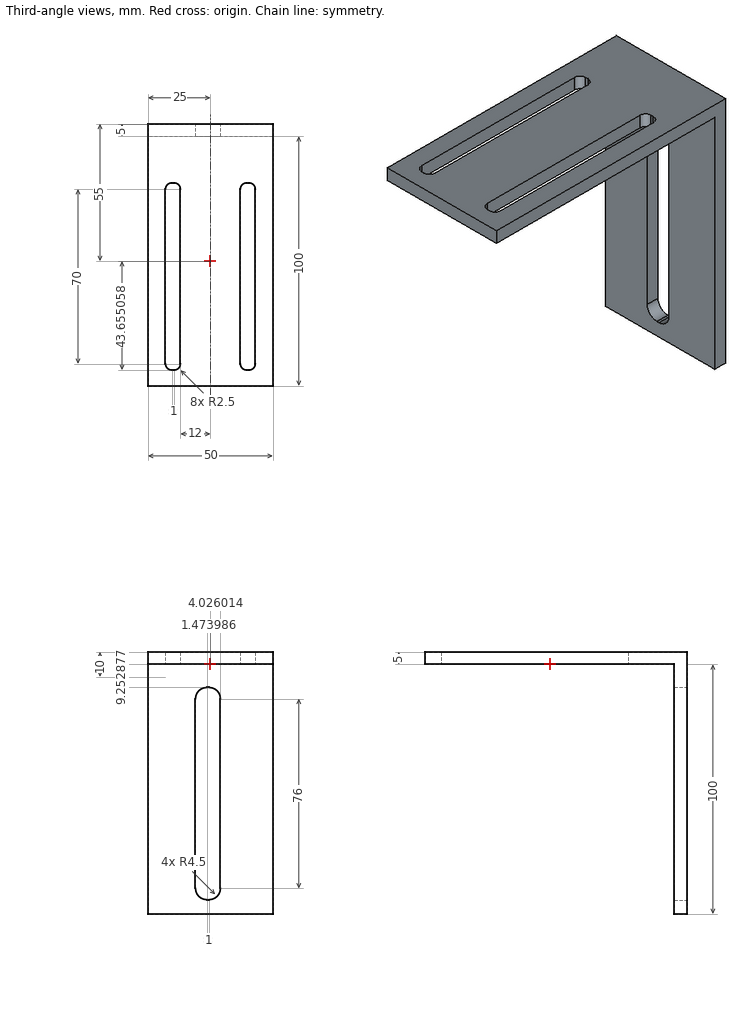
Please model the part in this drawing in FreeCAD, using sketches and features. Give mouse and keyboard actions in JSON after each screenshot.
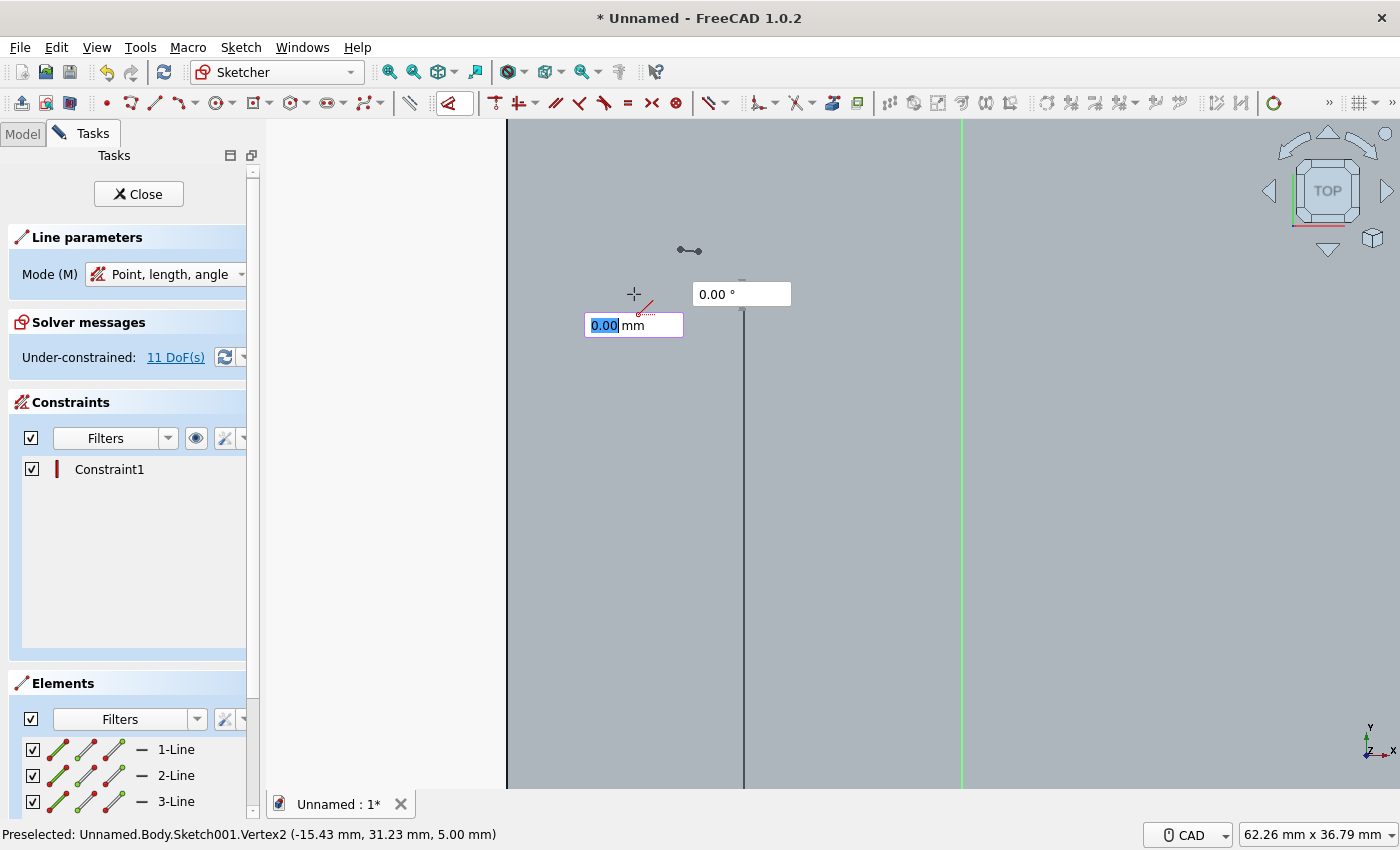
{"action": "scroll", "coordinate": [679, 248], "scroll_direction": "down", "scroll_amount": 6}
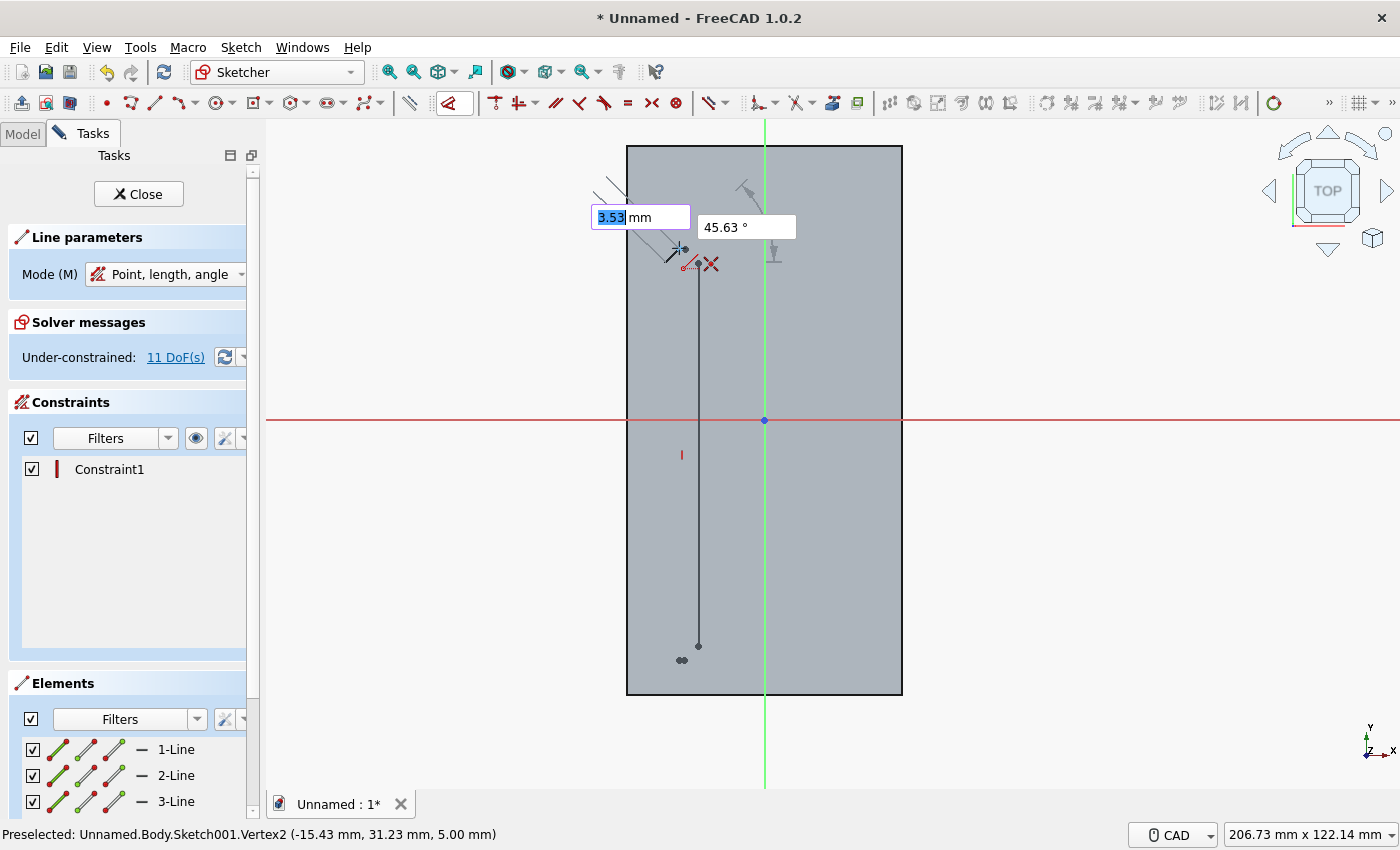
{"action": "left_click", "coordinate": [666, 646]}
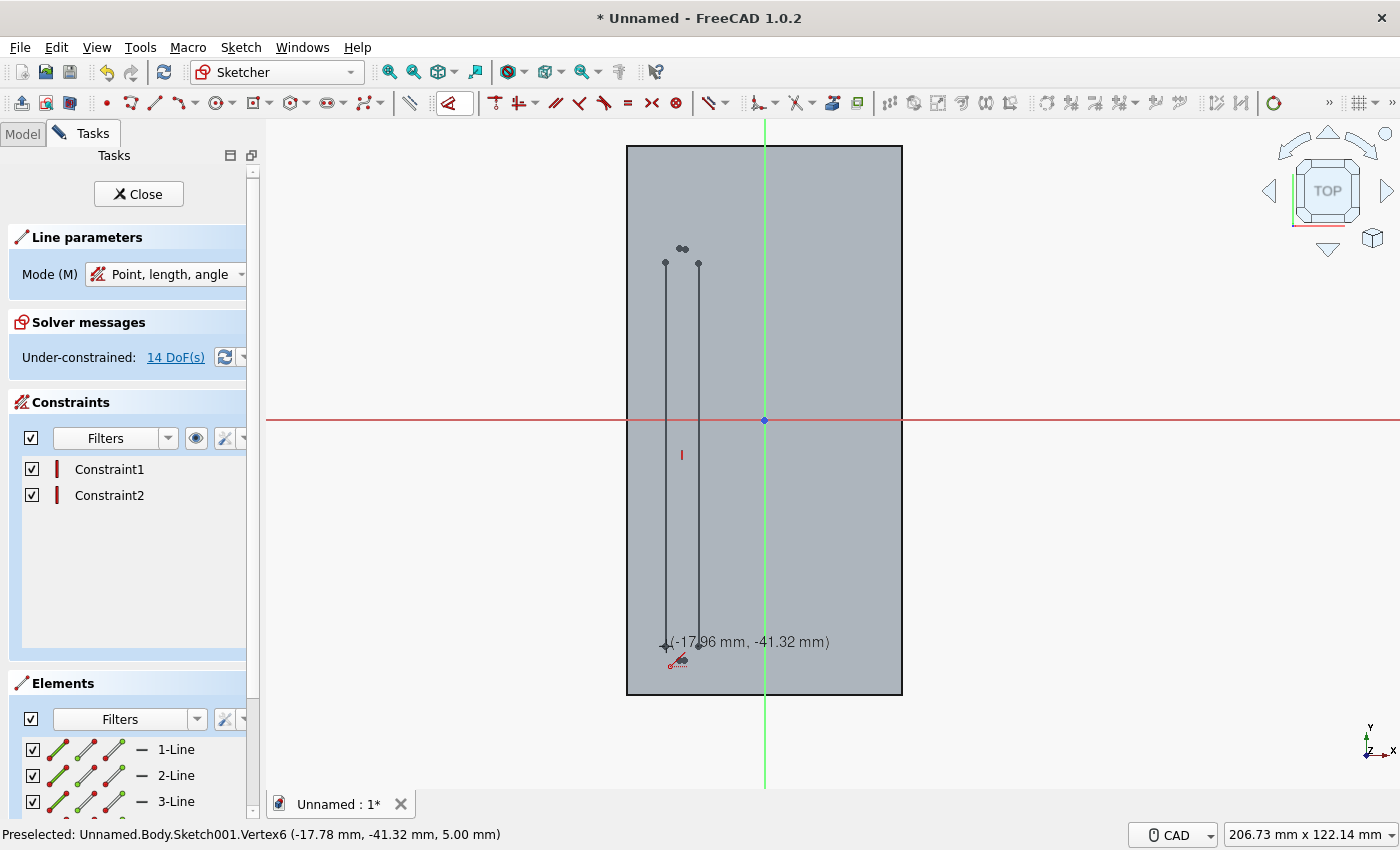
{"action": "key", "text": "g 3 a"}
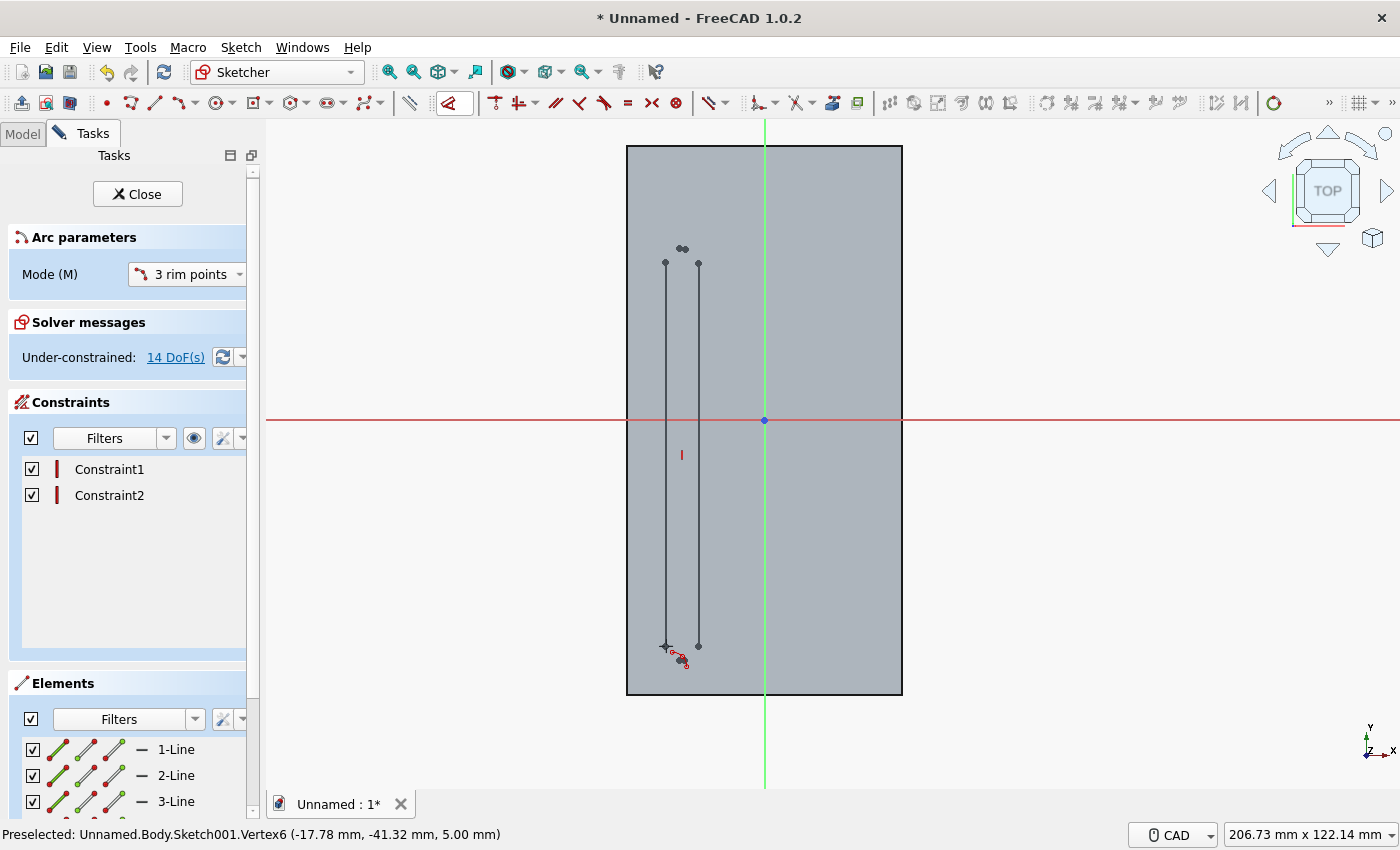
{"action": "scroll", "coordinate": [685, 660], "scroll_direction": "up", "scroll_amount": 9}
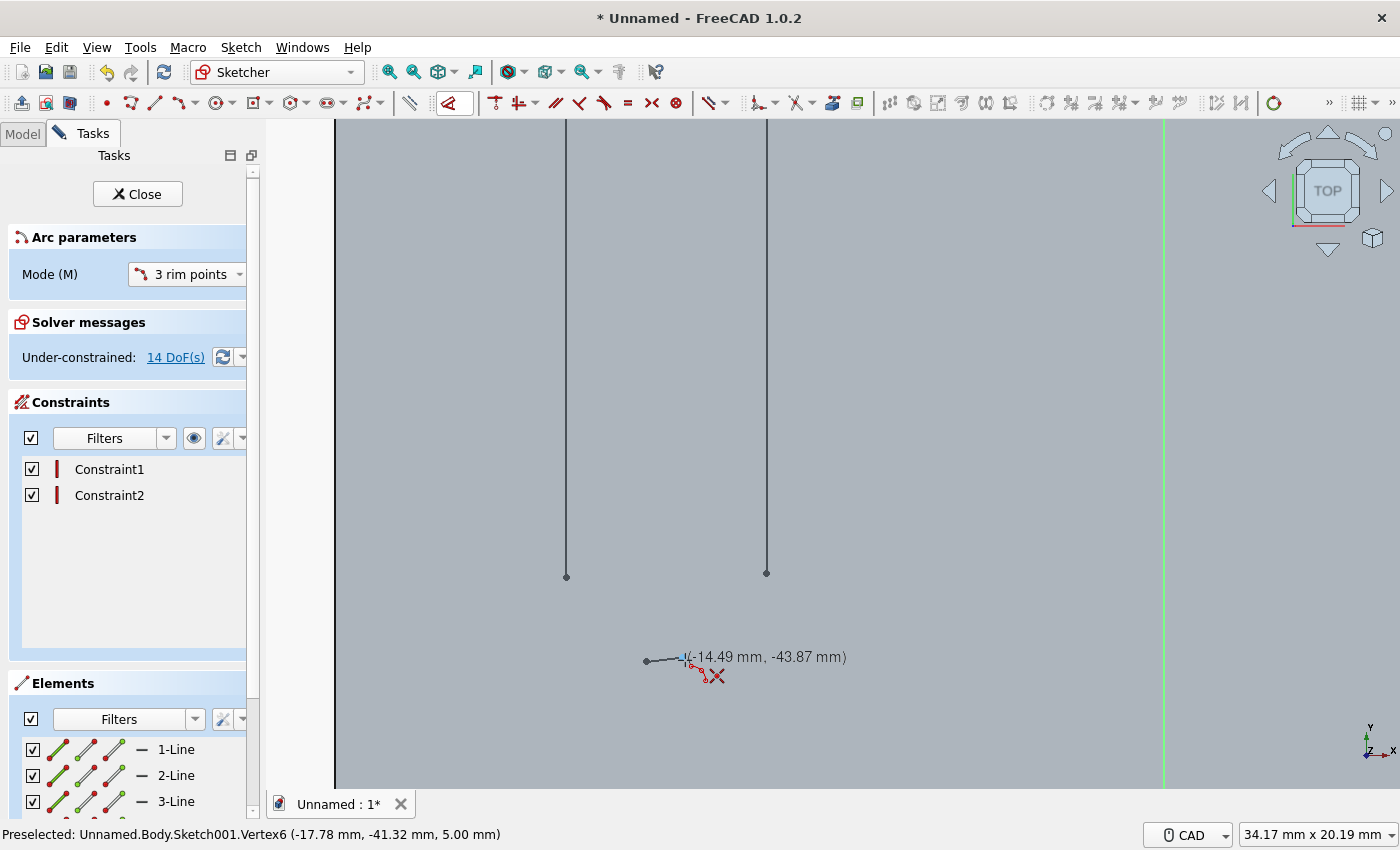
{"action": "left_click", "coordinate": [683, 658]}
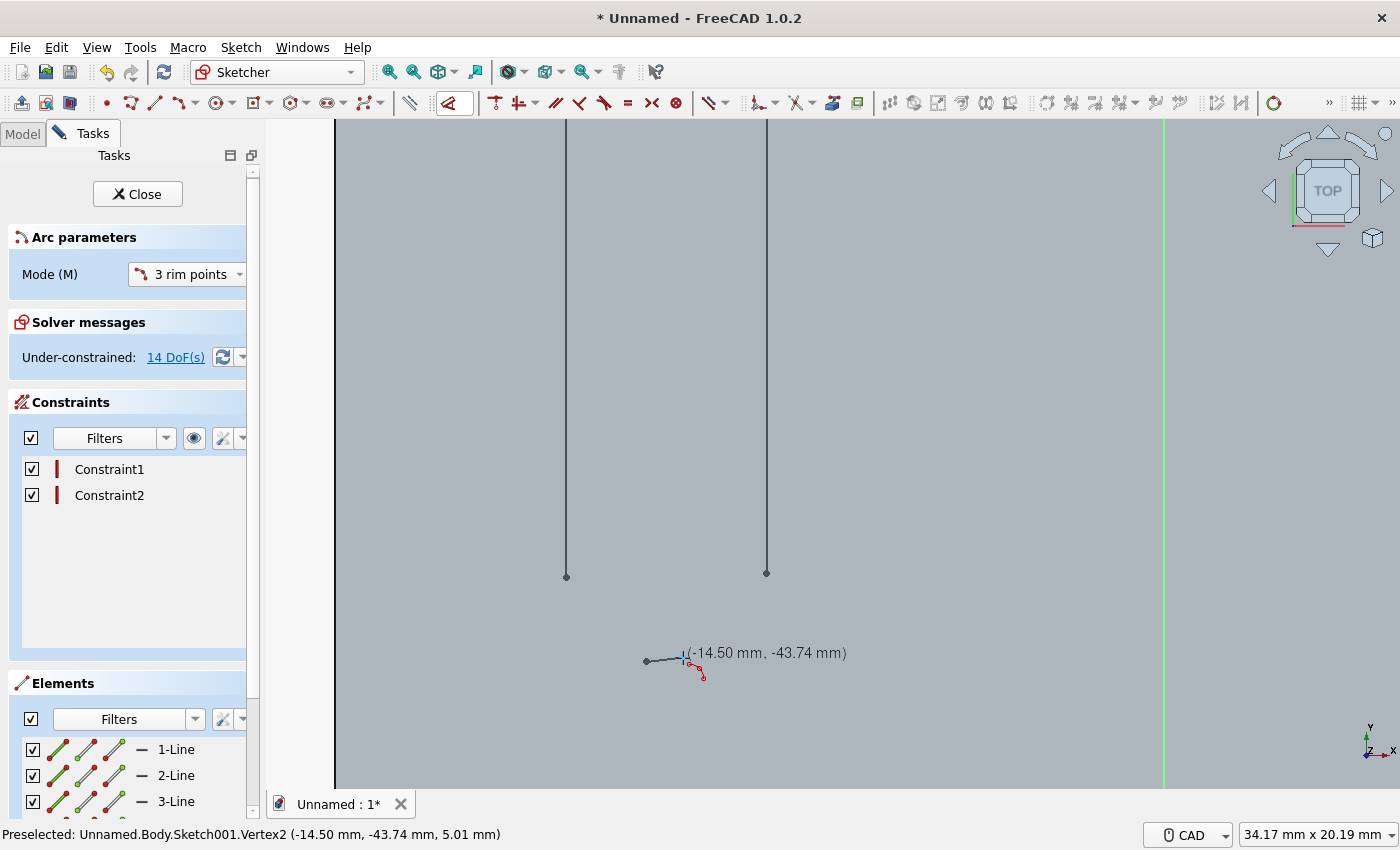
{"action": "scroll", "coordinate": [685, 661], "scroll_direction": "down", "scroll_amount": 9}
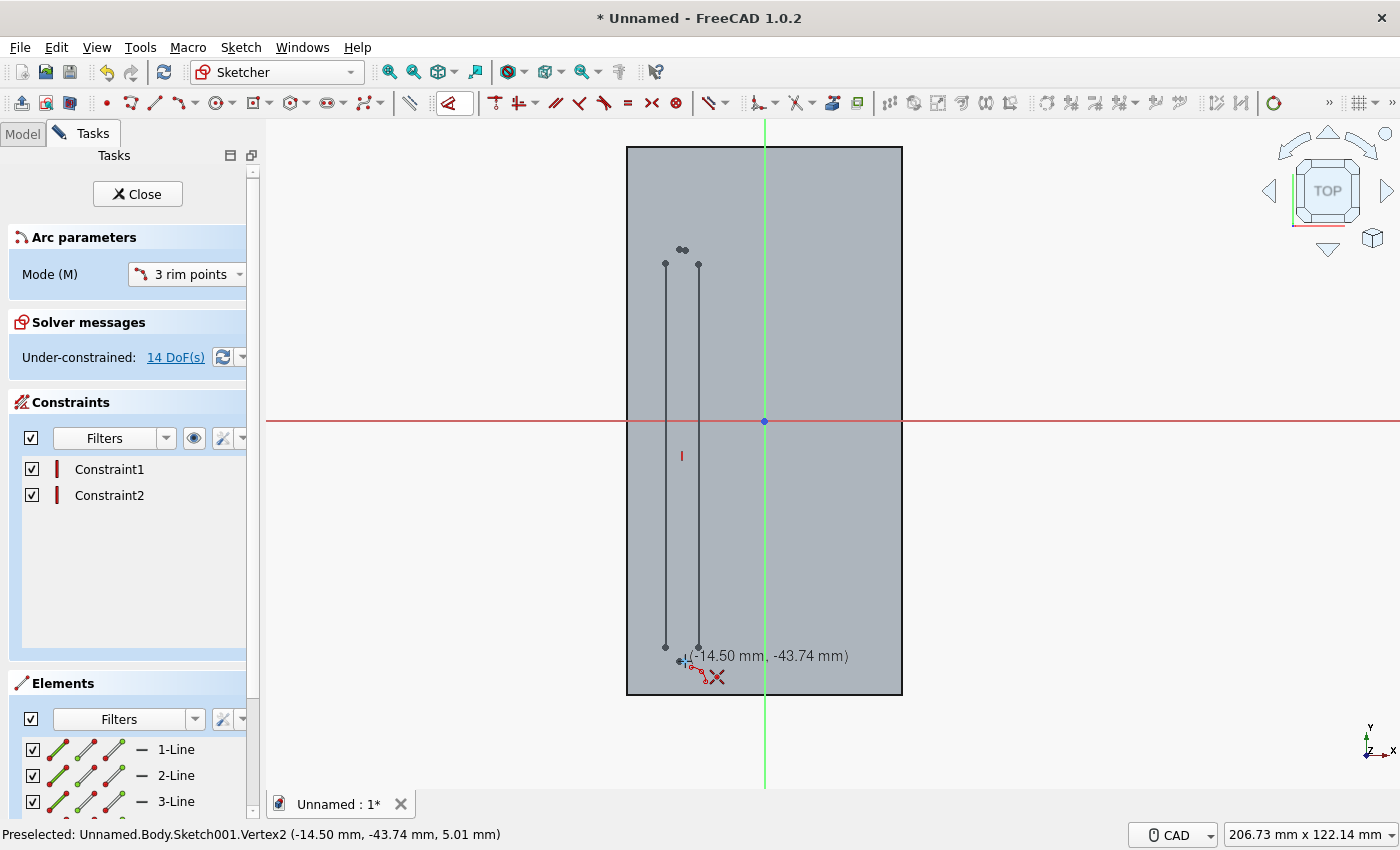
{"action": "left_click", "coordinate": [699, 647]}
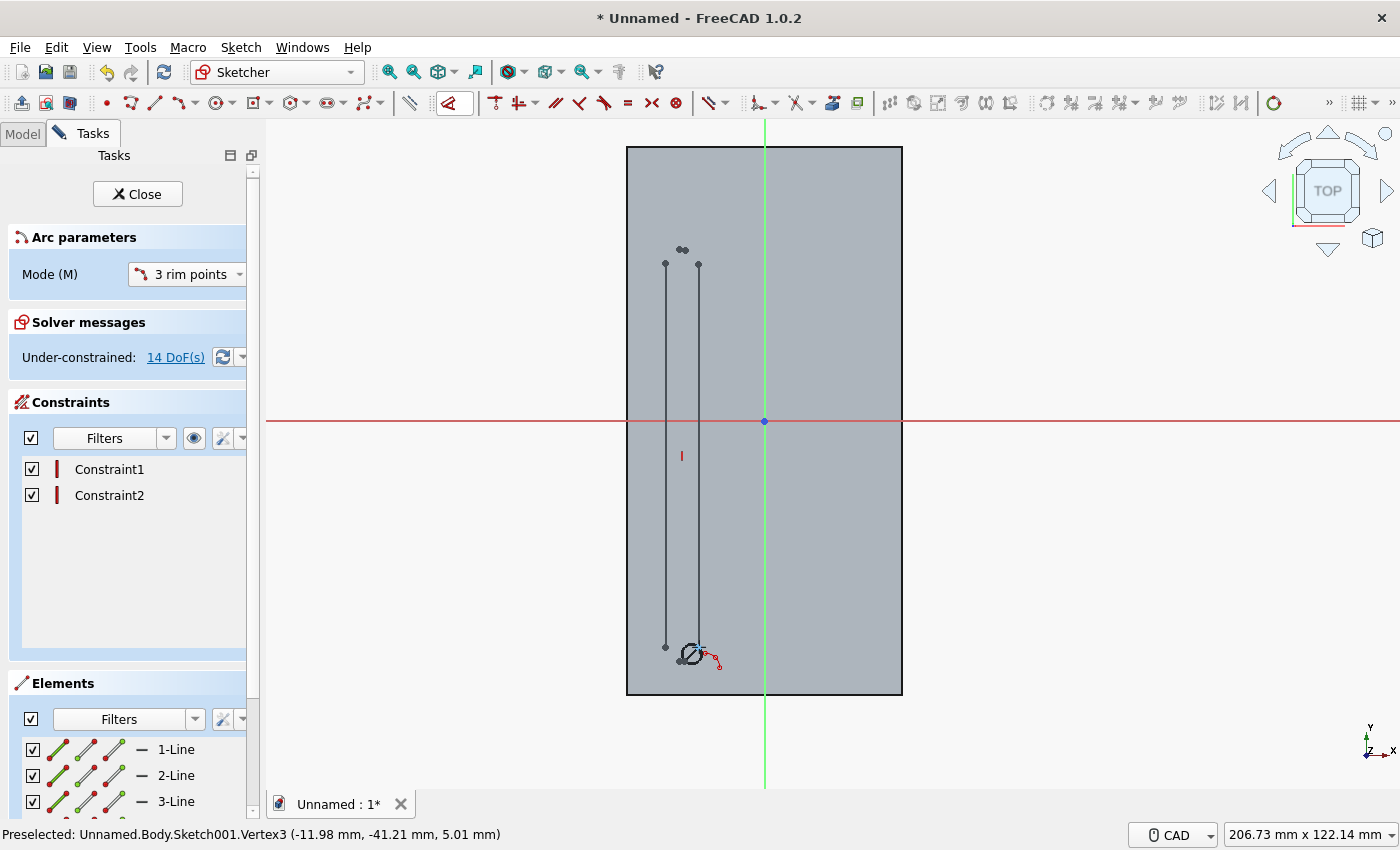
{"action": "scroll", "coordinate": [695, 657], "scroll_direction": "up", "scroll_amount": 7}